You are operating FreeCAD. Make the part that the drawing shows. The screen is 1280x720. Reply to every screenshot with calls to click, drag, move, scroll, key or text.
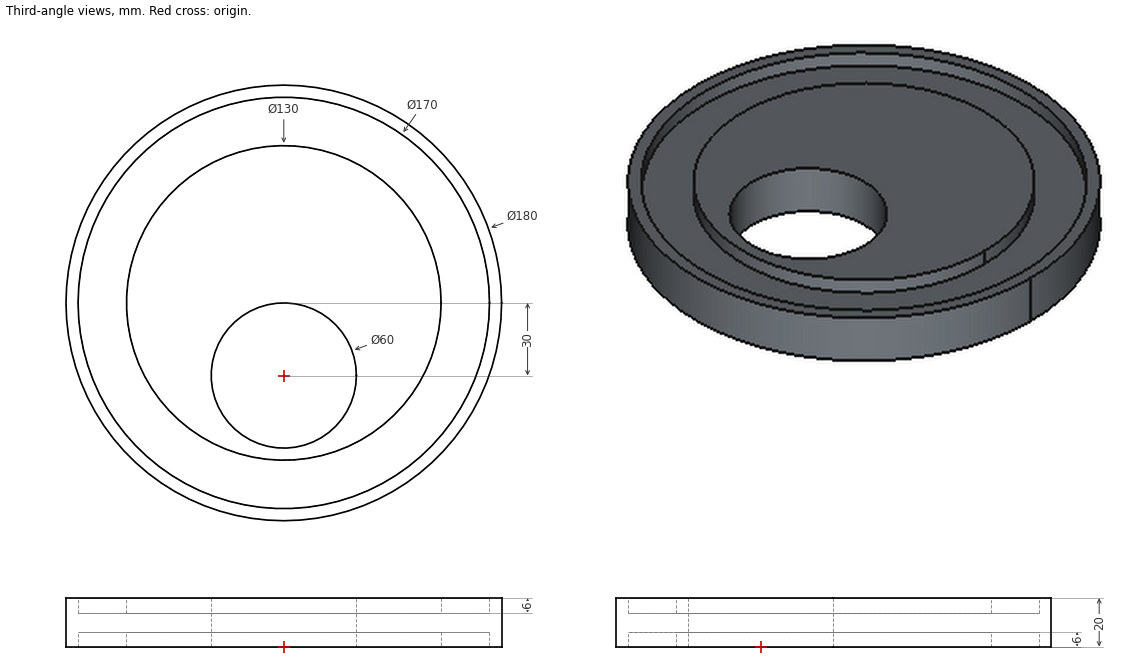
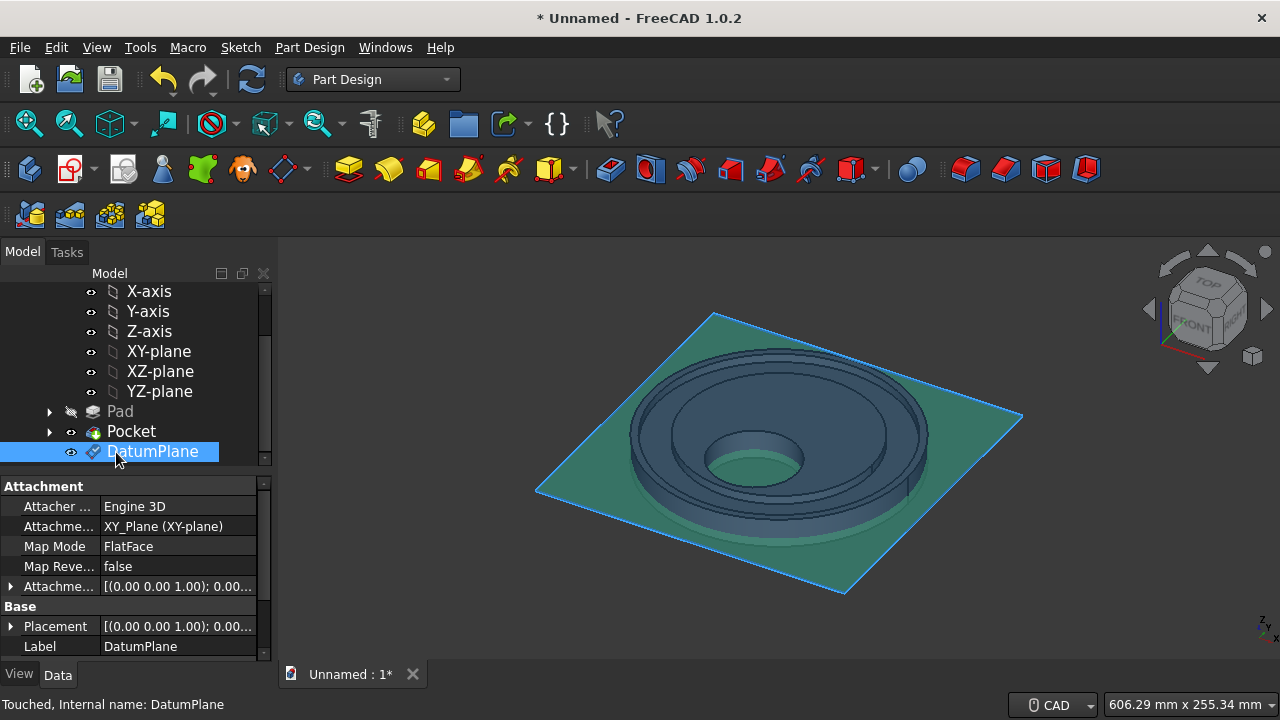
click(70, 170)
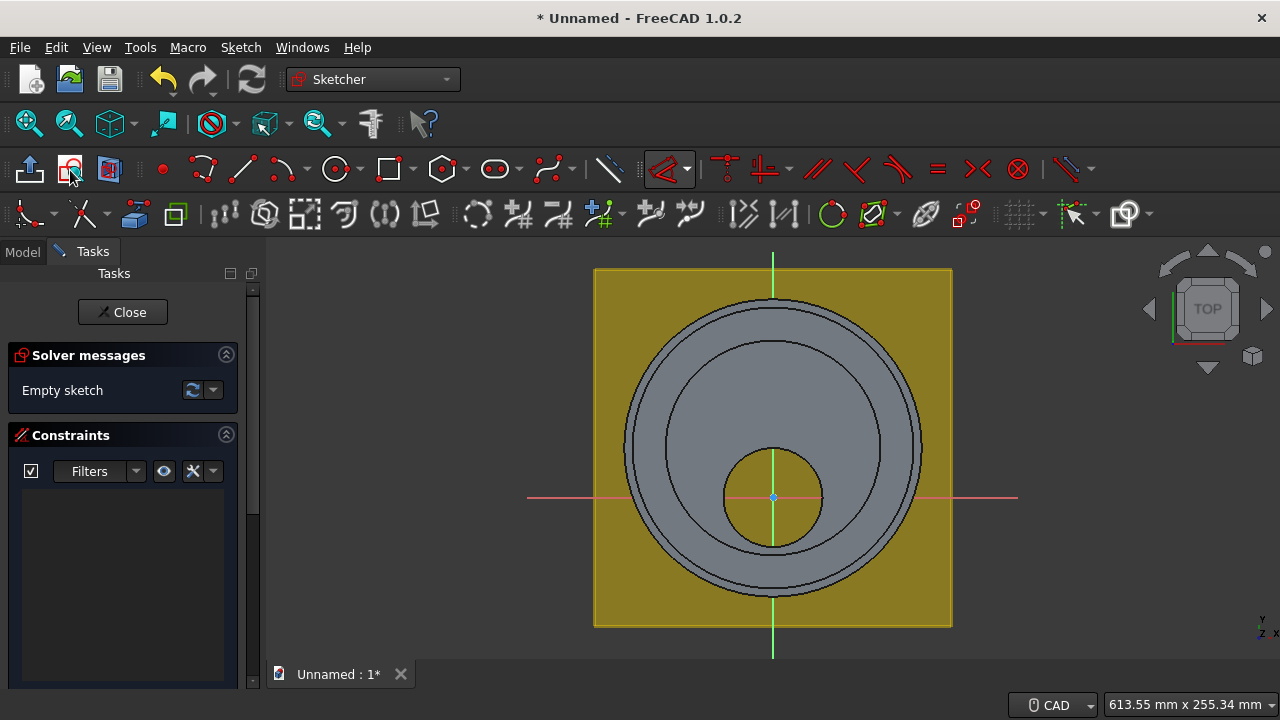
click(110, 170)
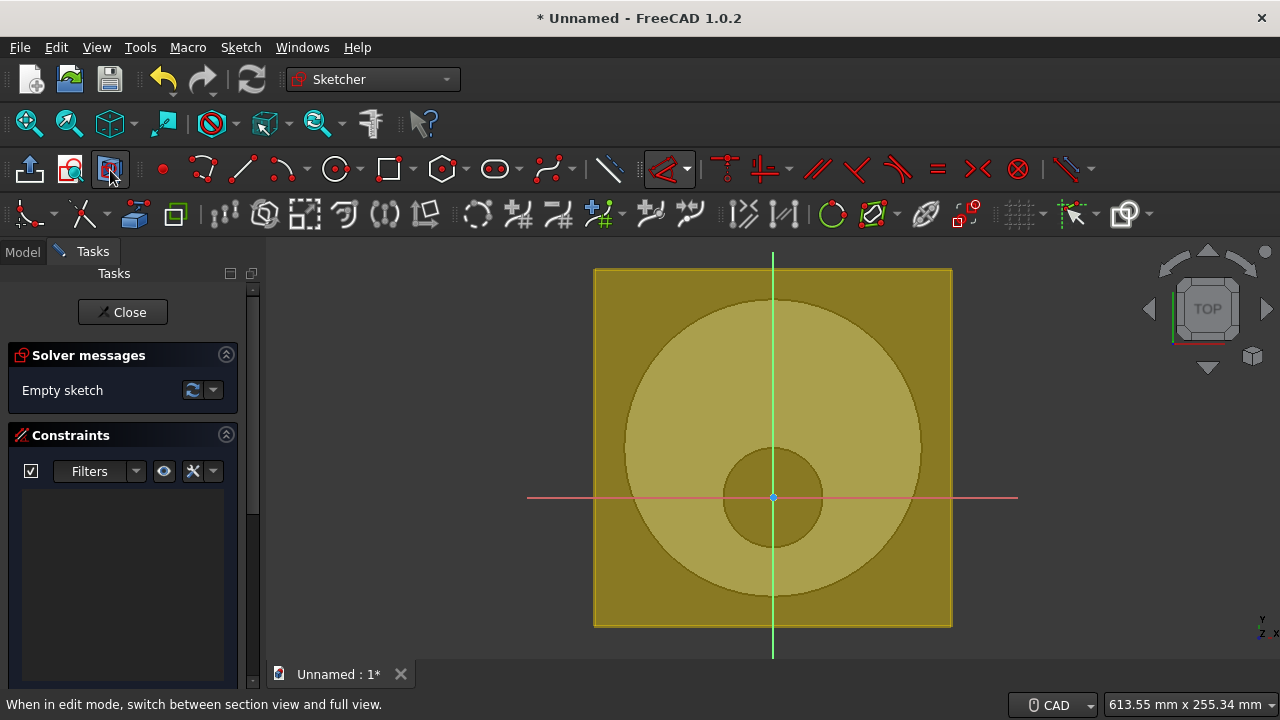
click(336, 170)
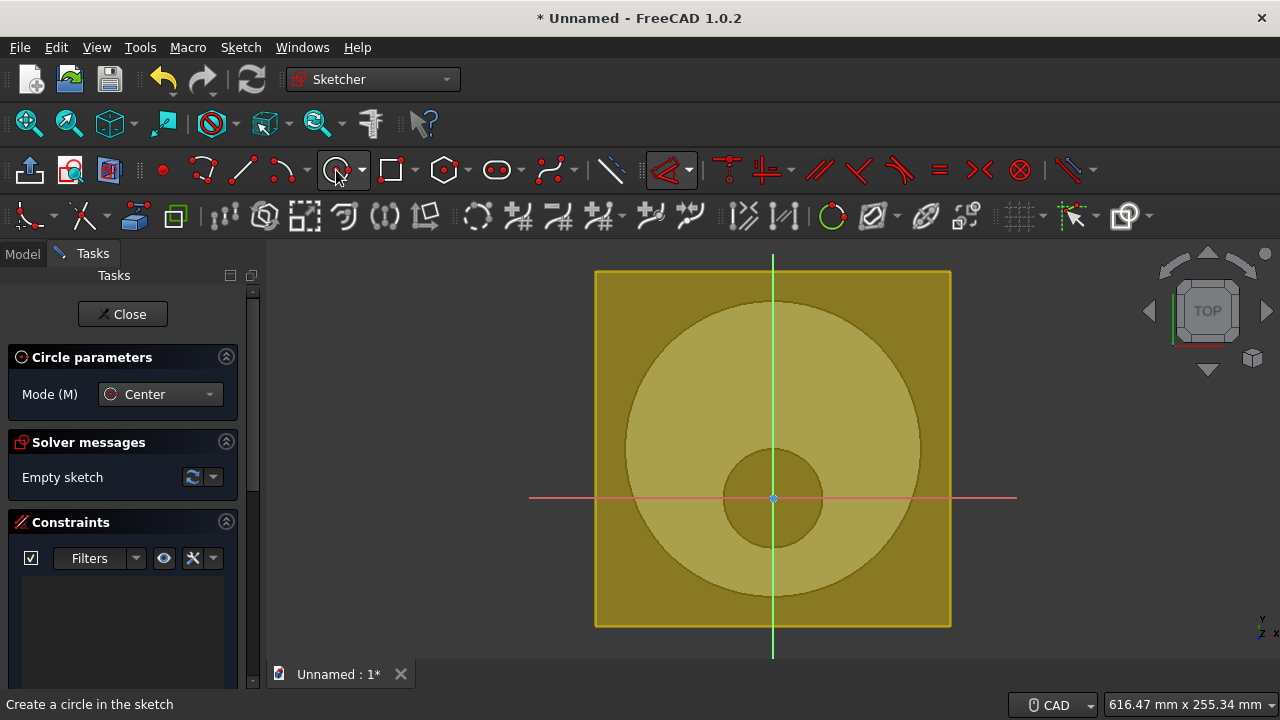
click(773, 449)
move(872, 350)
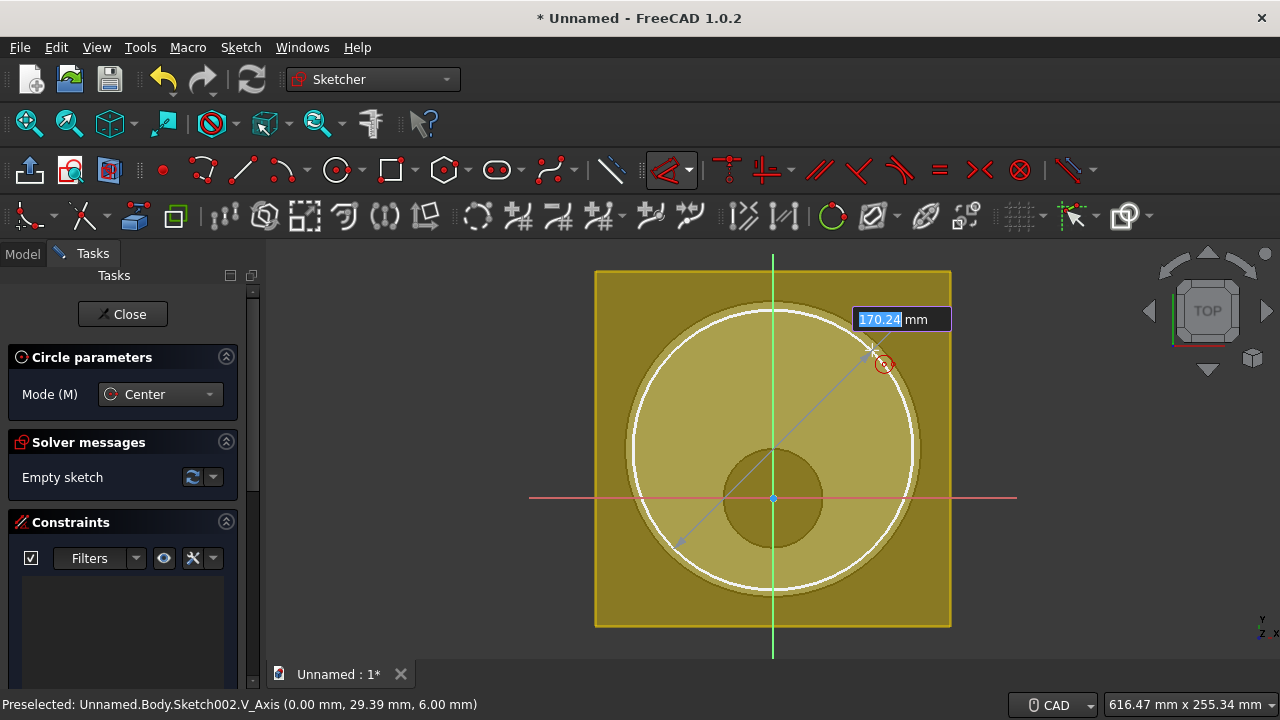
text(170)
key(Return)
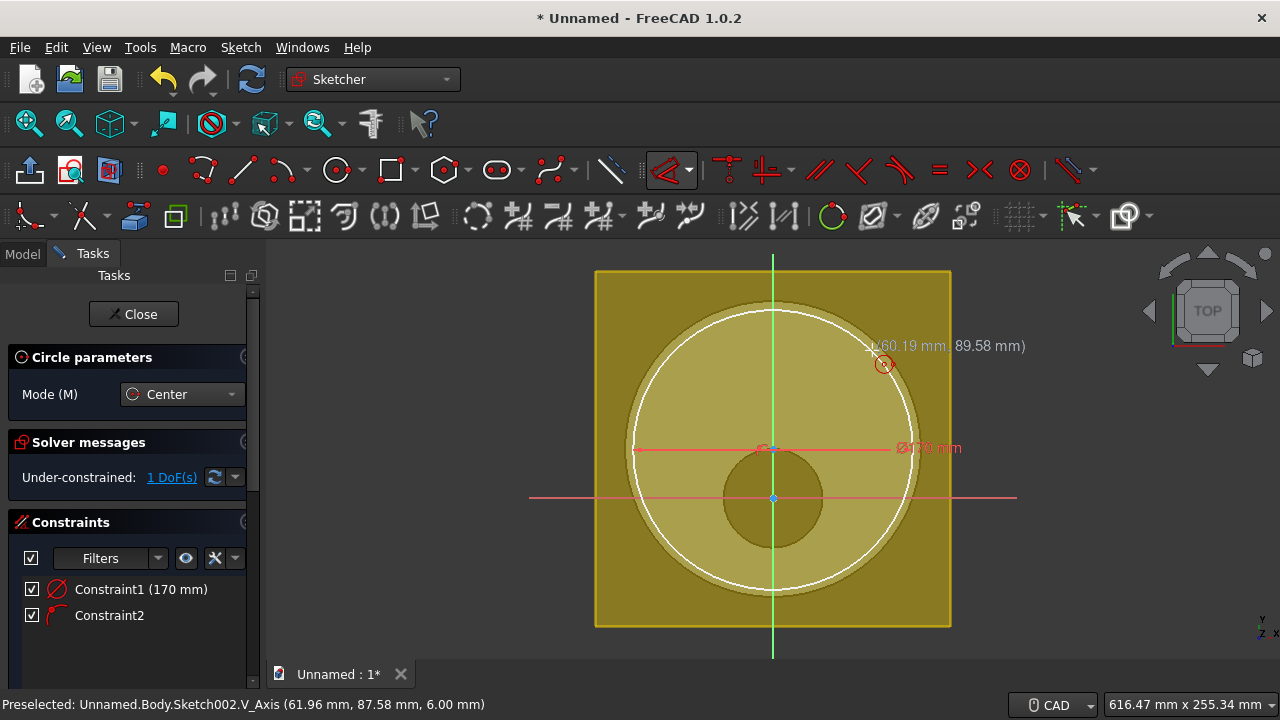
click(773, 450)
move(849, 373)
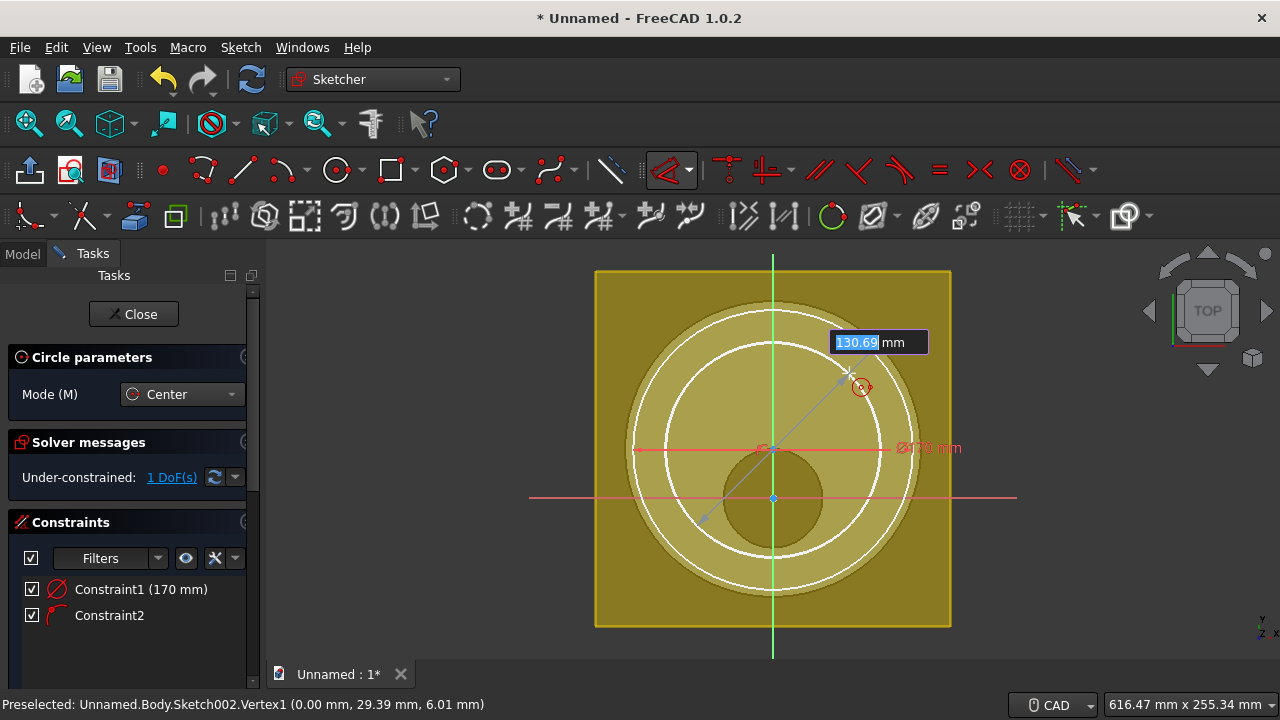
text(130)
key(Return)
key(Escape)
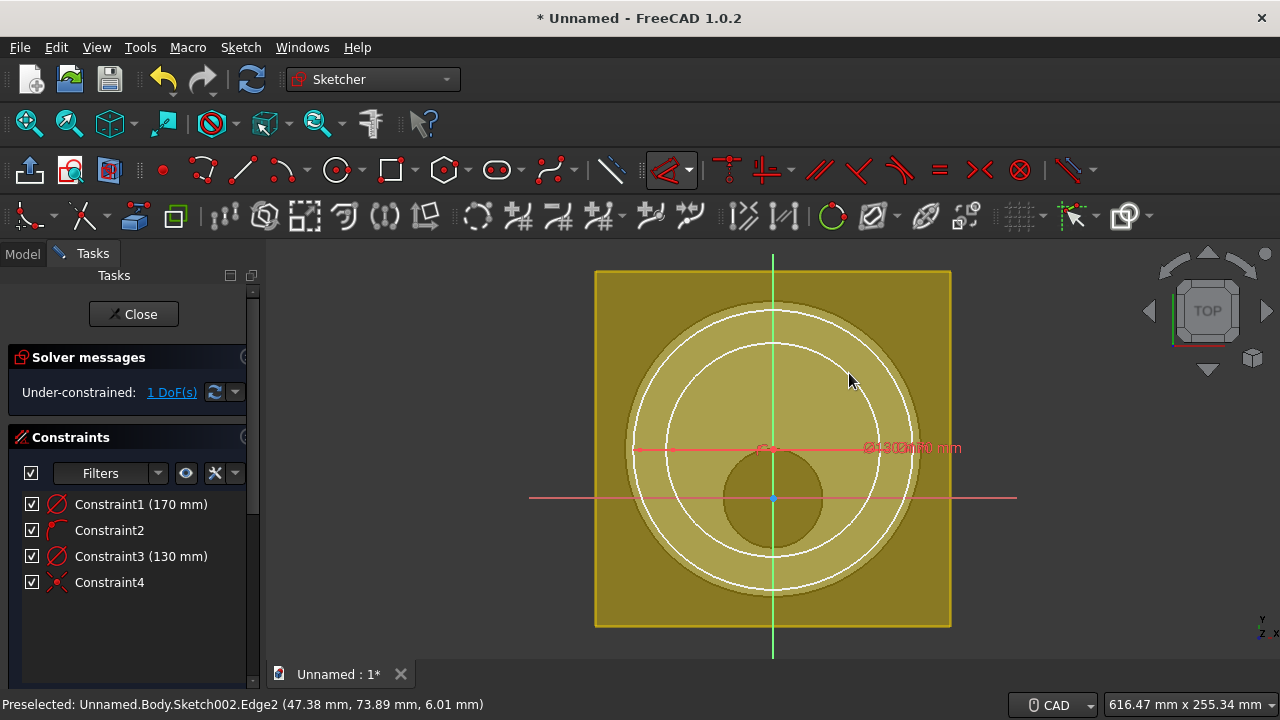
click(773, 450)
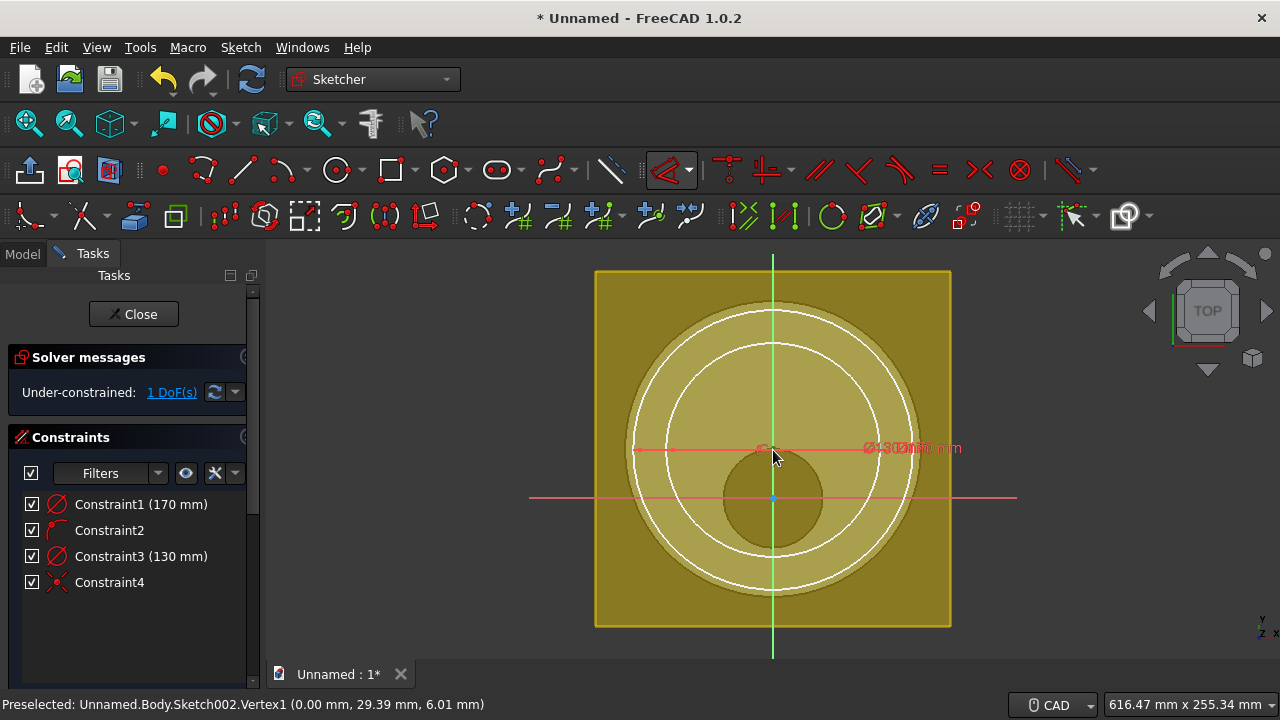
key(i)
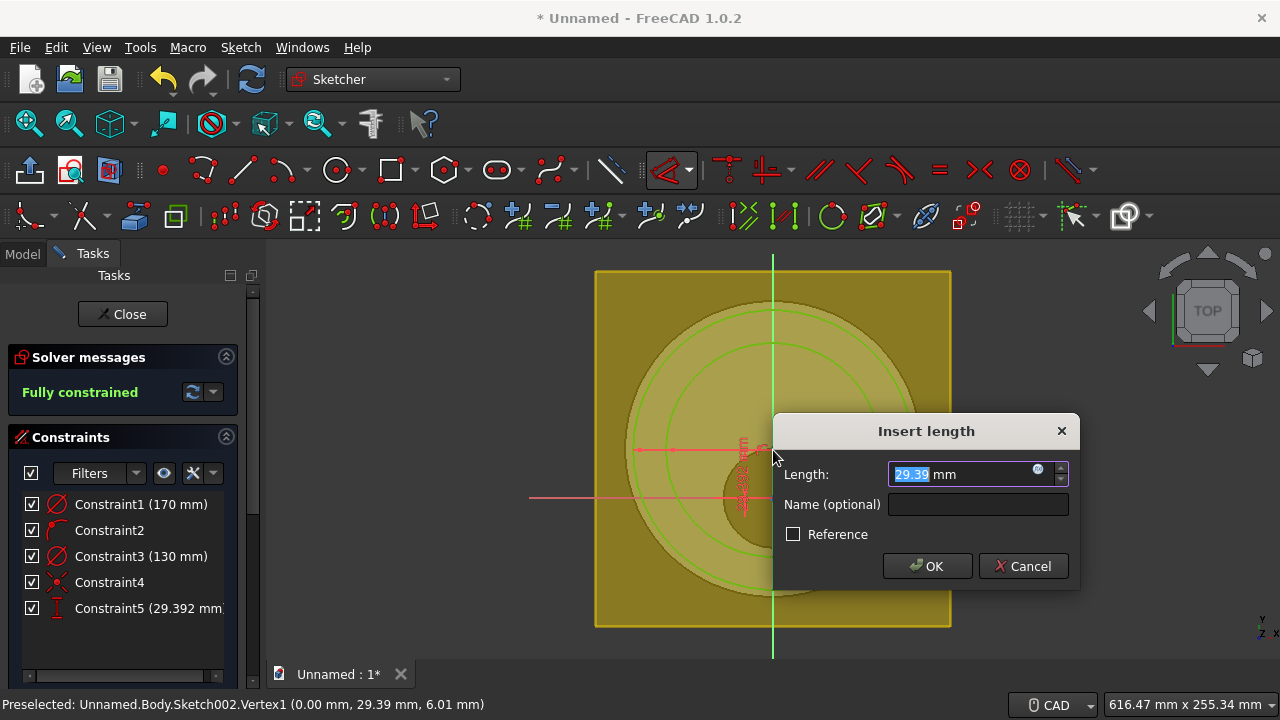
text(30)
key(Return)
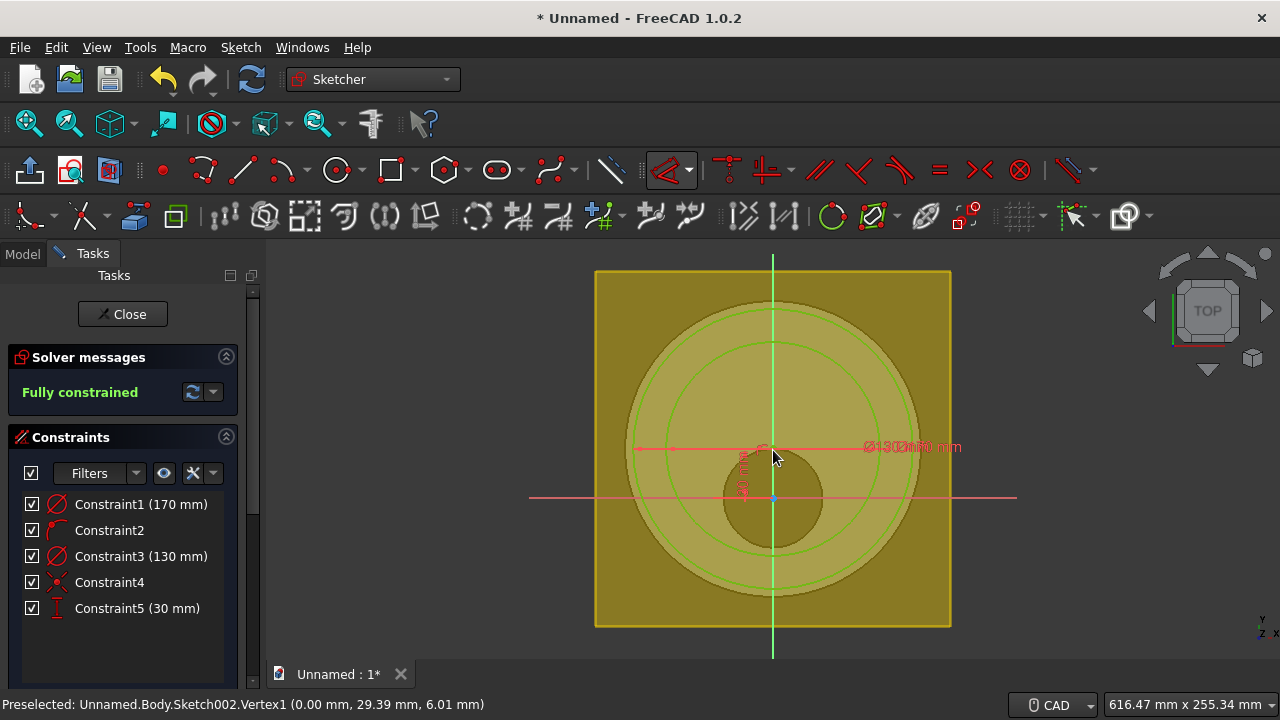
click(123, 314)